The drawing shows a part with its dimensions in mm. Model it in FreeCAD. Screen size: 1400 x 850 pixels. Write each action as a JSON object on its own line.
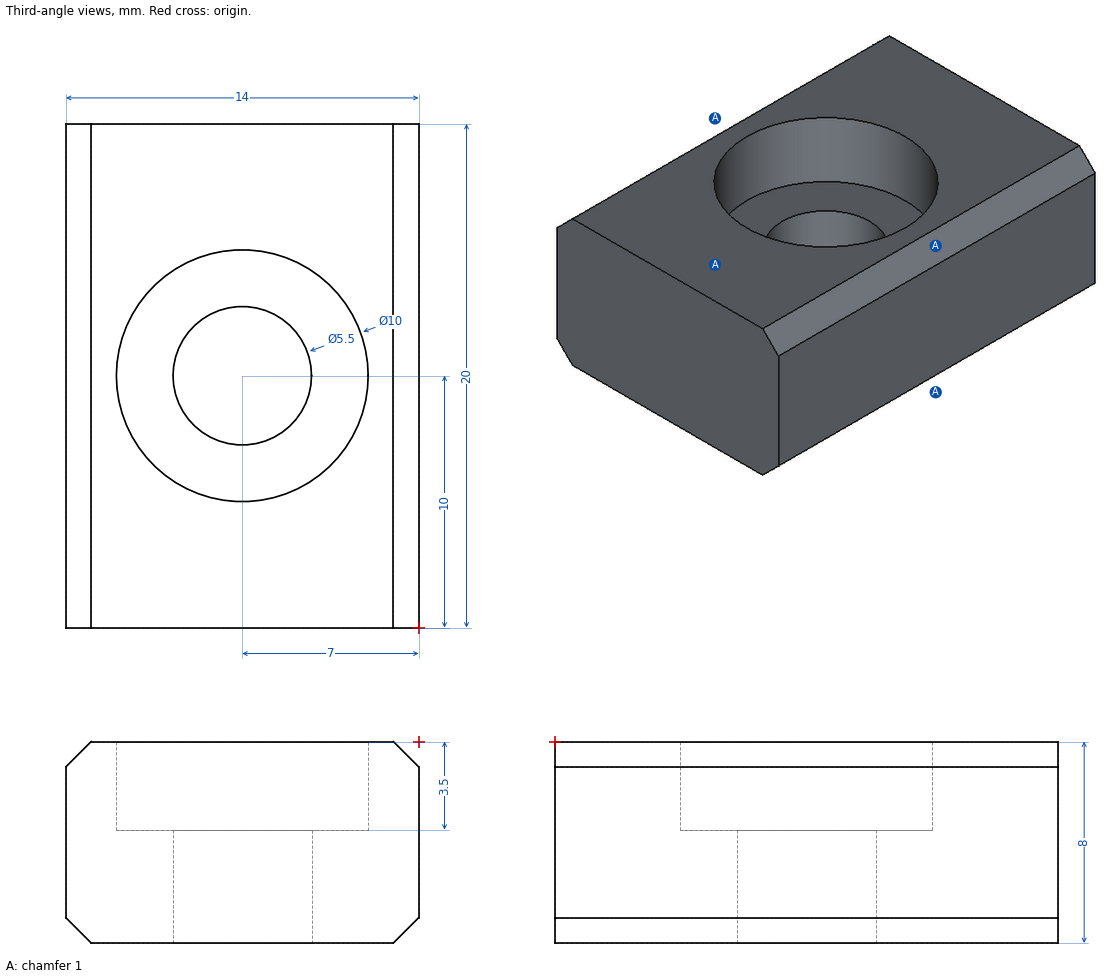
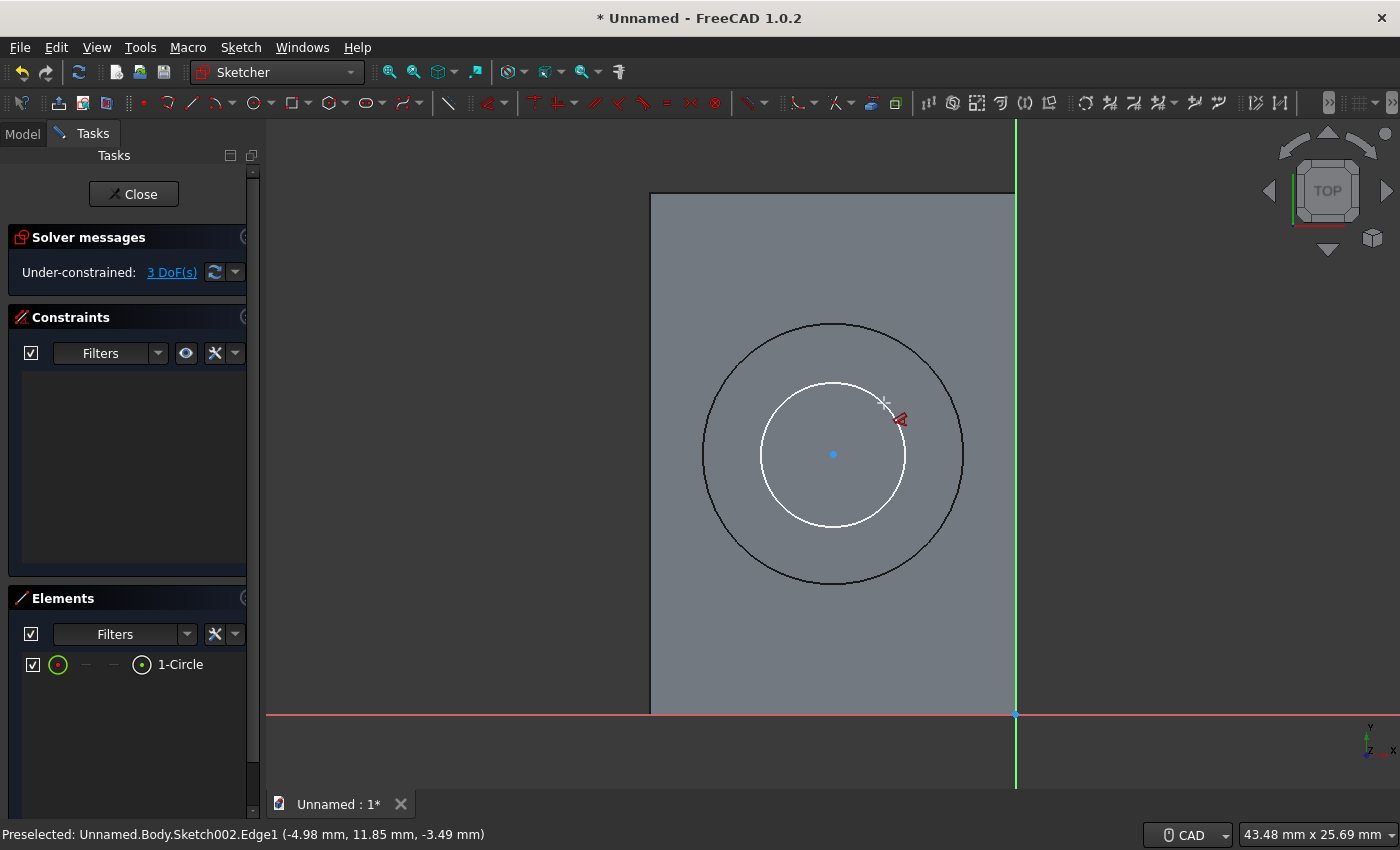
{"action": "left_click", "coordinate": [884, 404]}
{"action": "left_click", "coordinate": [907, 381]}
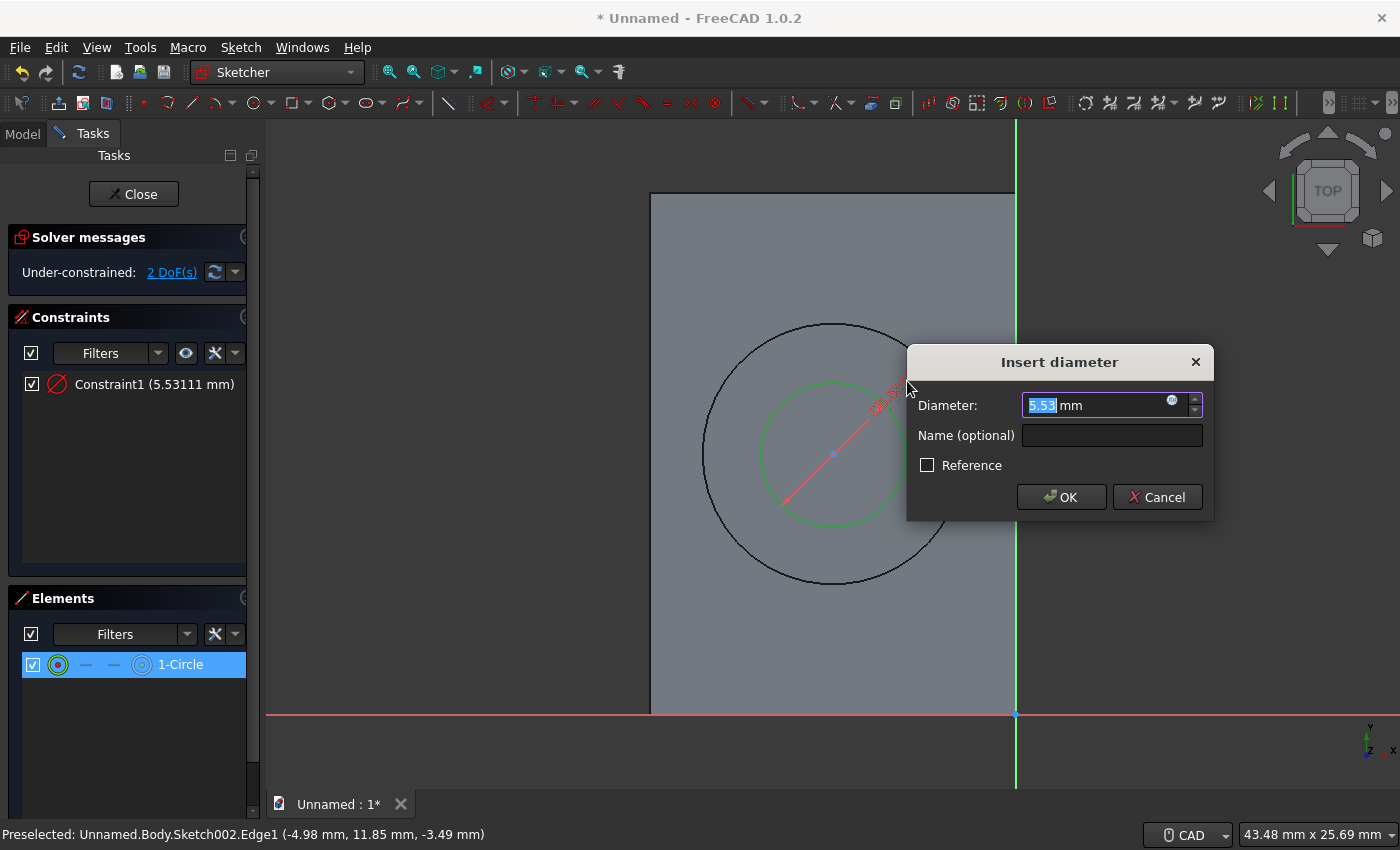
{"action": "type", "text": "5.5"}
{"action": "key", "text": "Return"}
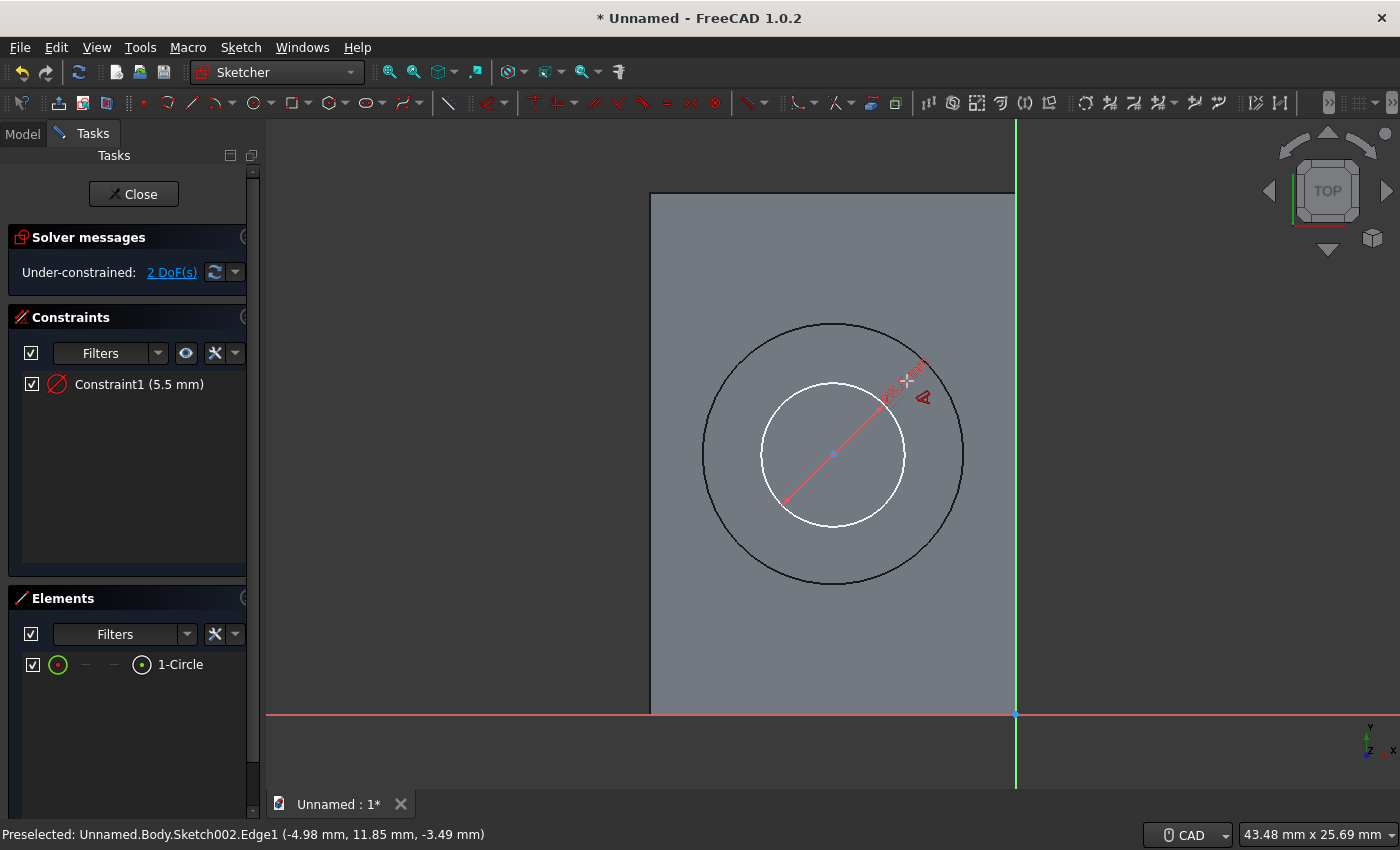
{"action": "left_click", "coordinate": [833, 455]}
{"action": "left_click", "coordinate": [924, 749]}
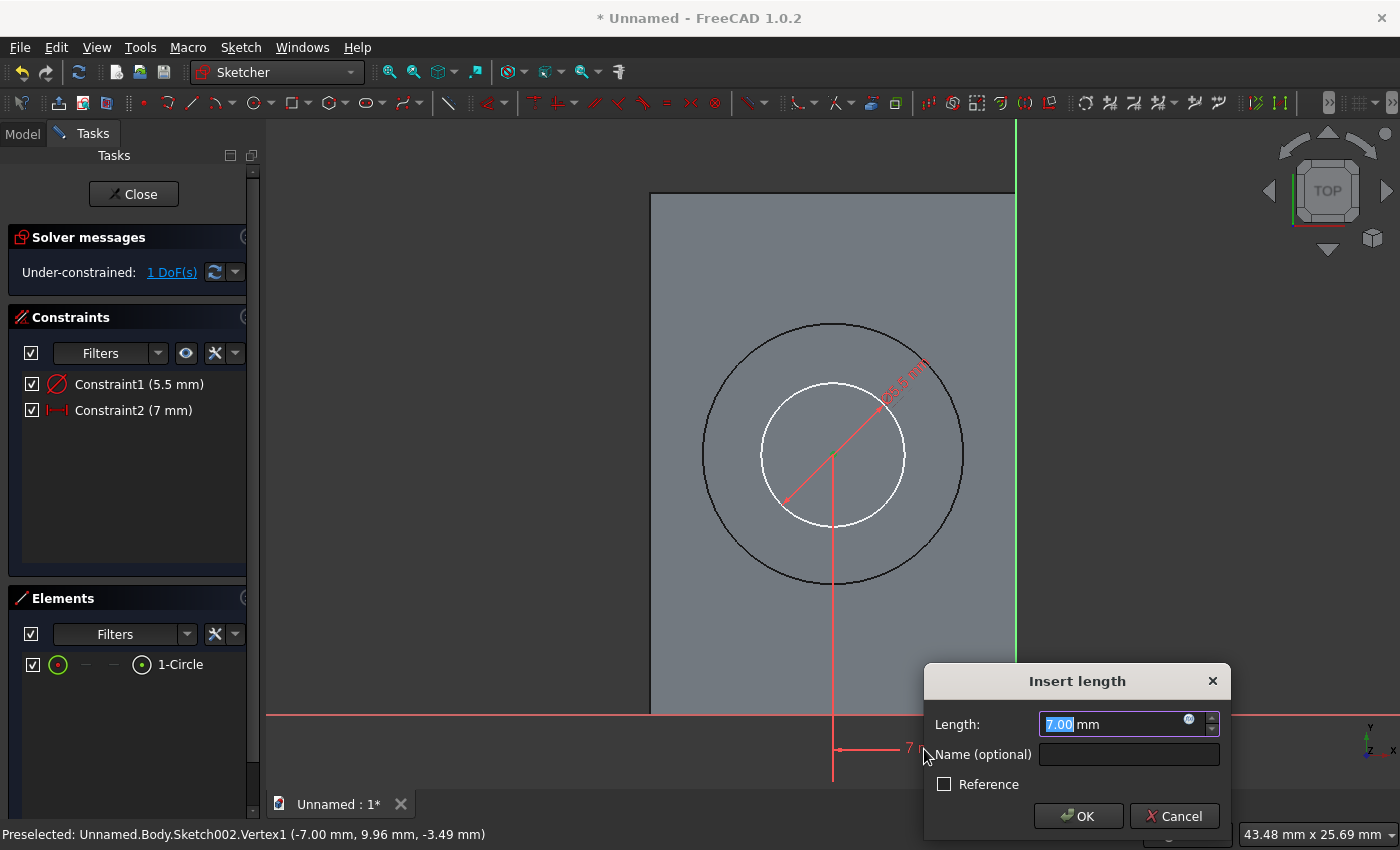
{"action": "type", "text": "7"}
{"action": "key", "text": "Return"}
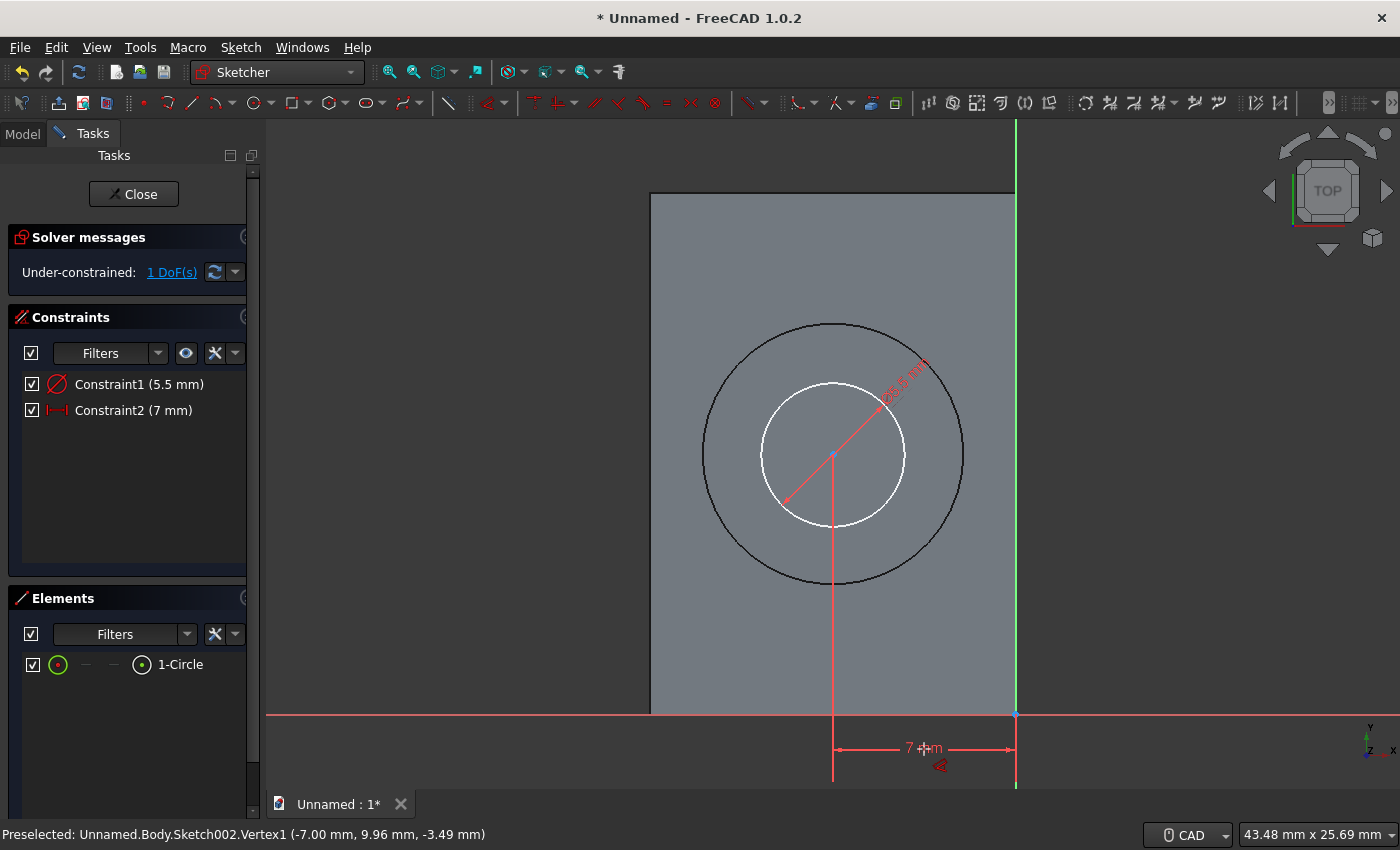
{"action": "left_click", "coordinate": [833, 455]}
{"action": "left_click", "coordinate": [1050, 585]}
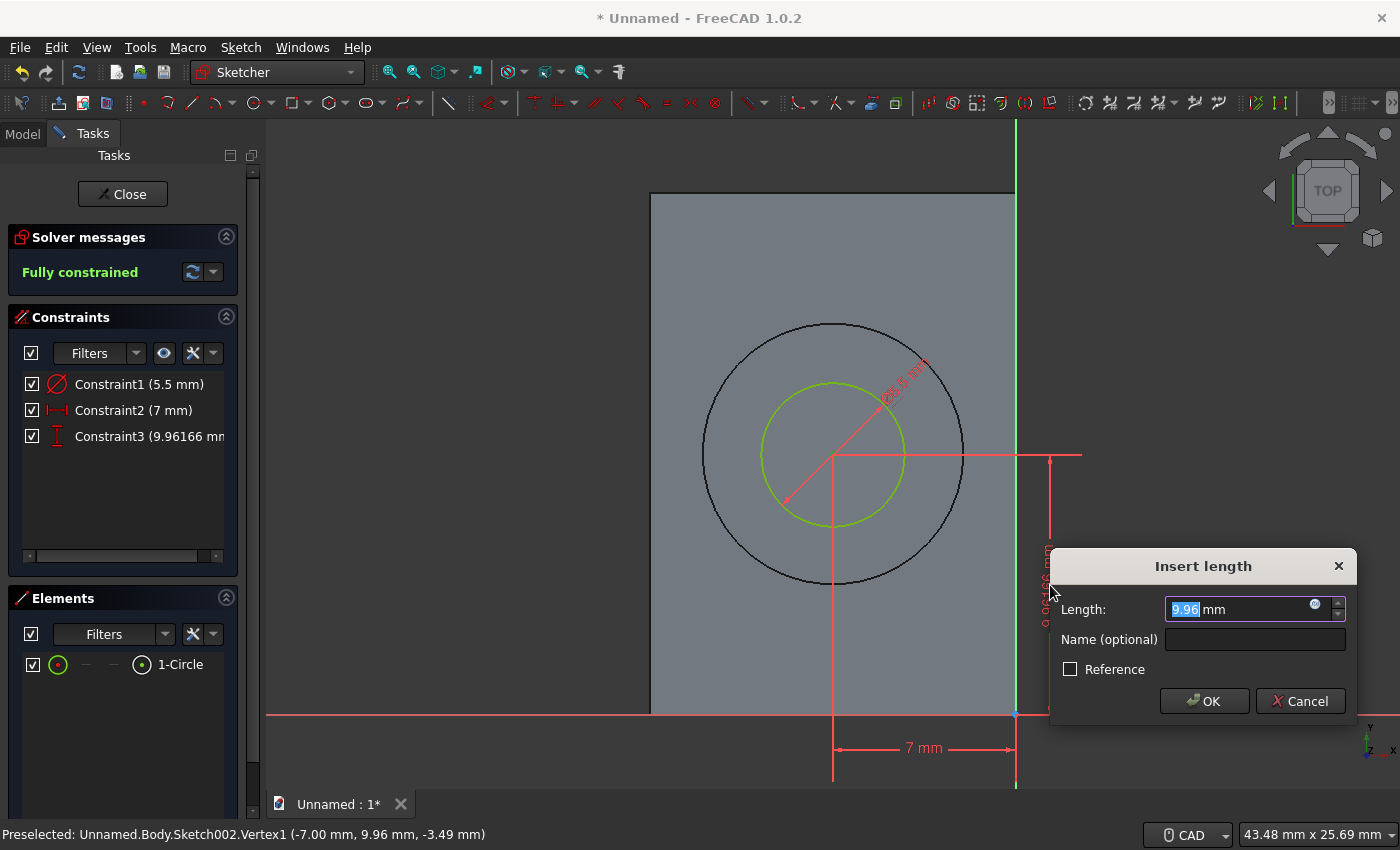
{"action": "type", "text": "10"}
{"action": "key", "text": "Return"}
{"action": "key", "text": "Escape"}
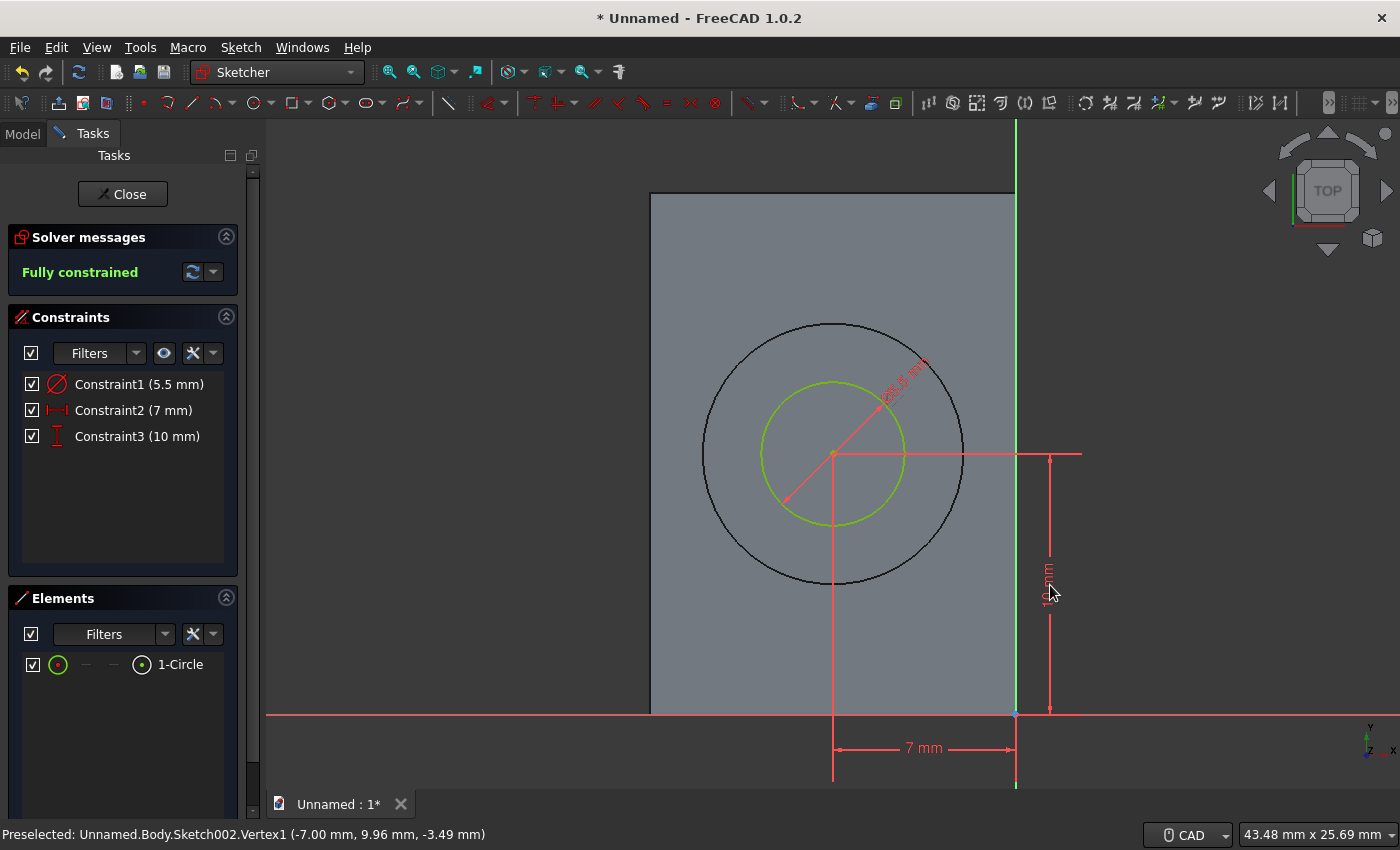
{"action": "left_click", "coordinate": [123, 194]}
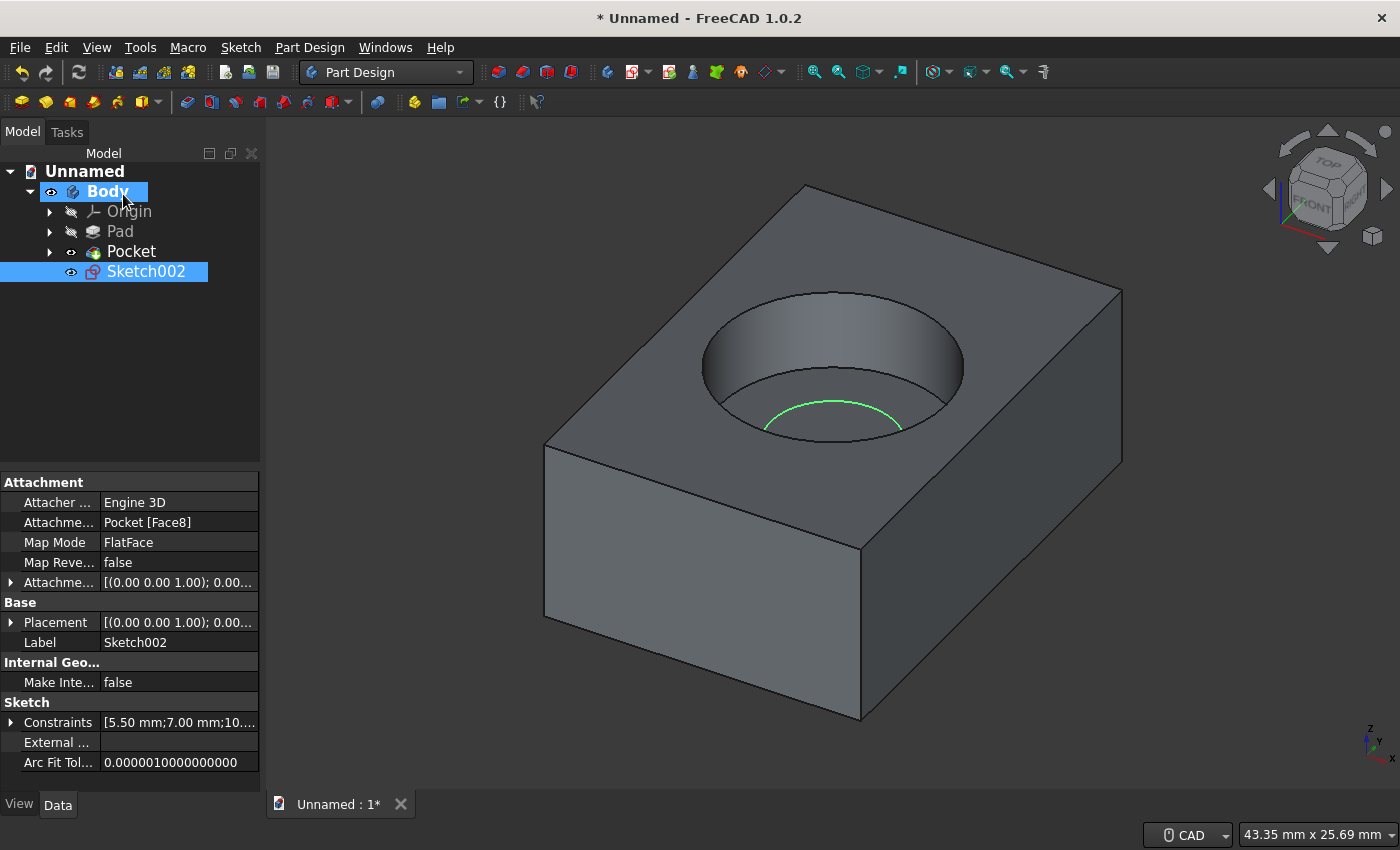
{"action": "left_click", "coordinate": [188, 102]}